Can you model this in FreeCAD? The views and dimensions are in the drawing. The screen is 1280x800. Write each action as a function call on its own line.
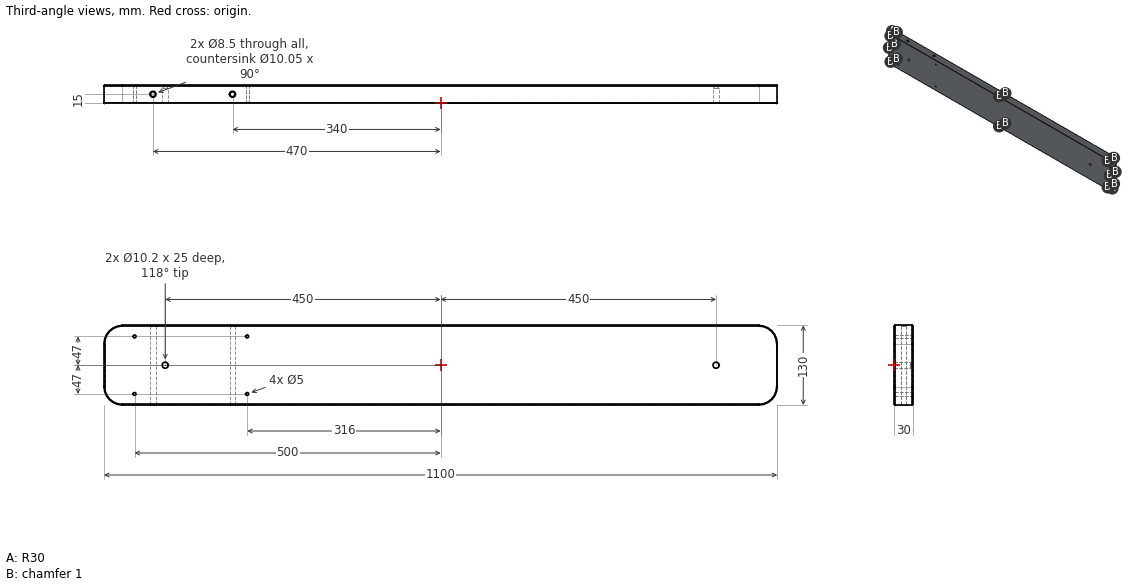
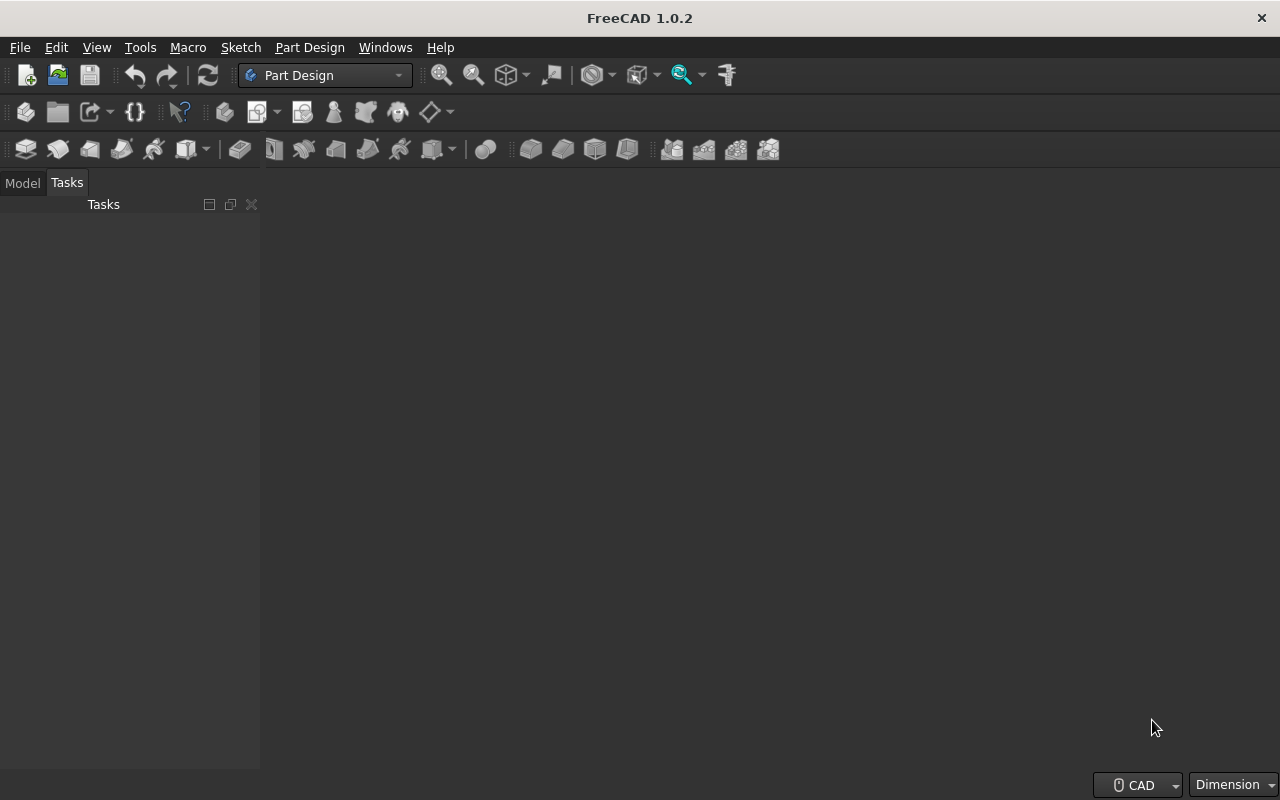
click(26, 76)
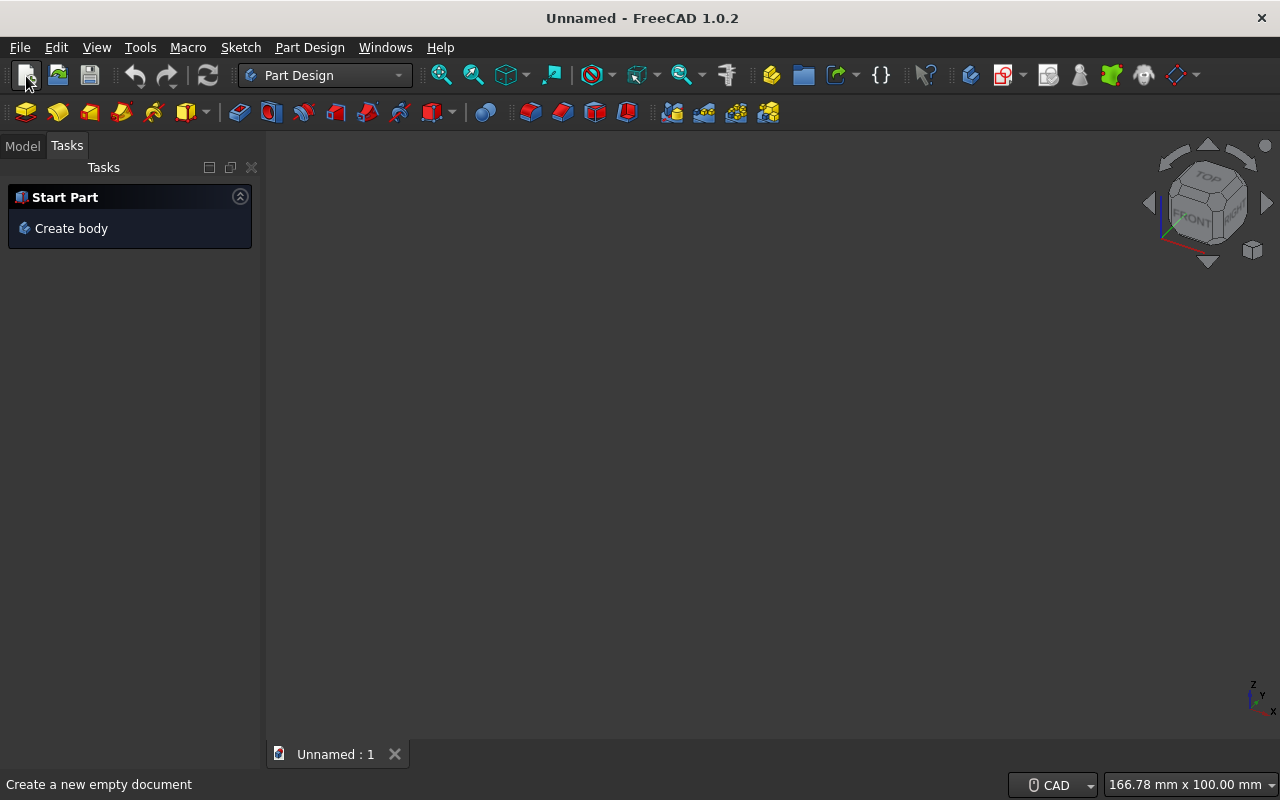
click(1004, 76)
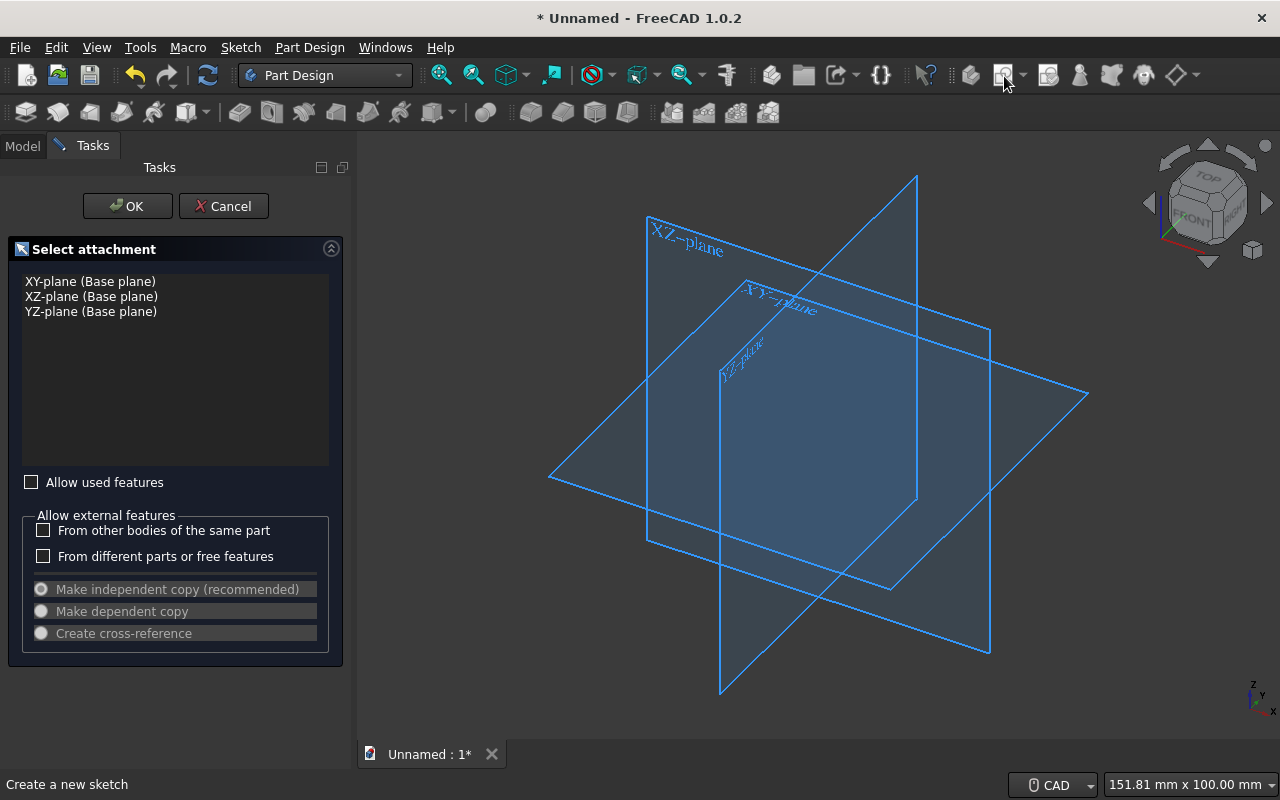
click(82, 296)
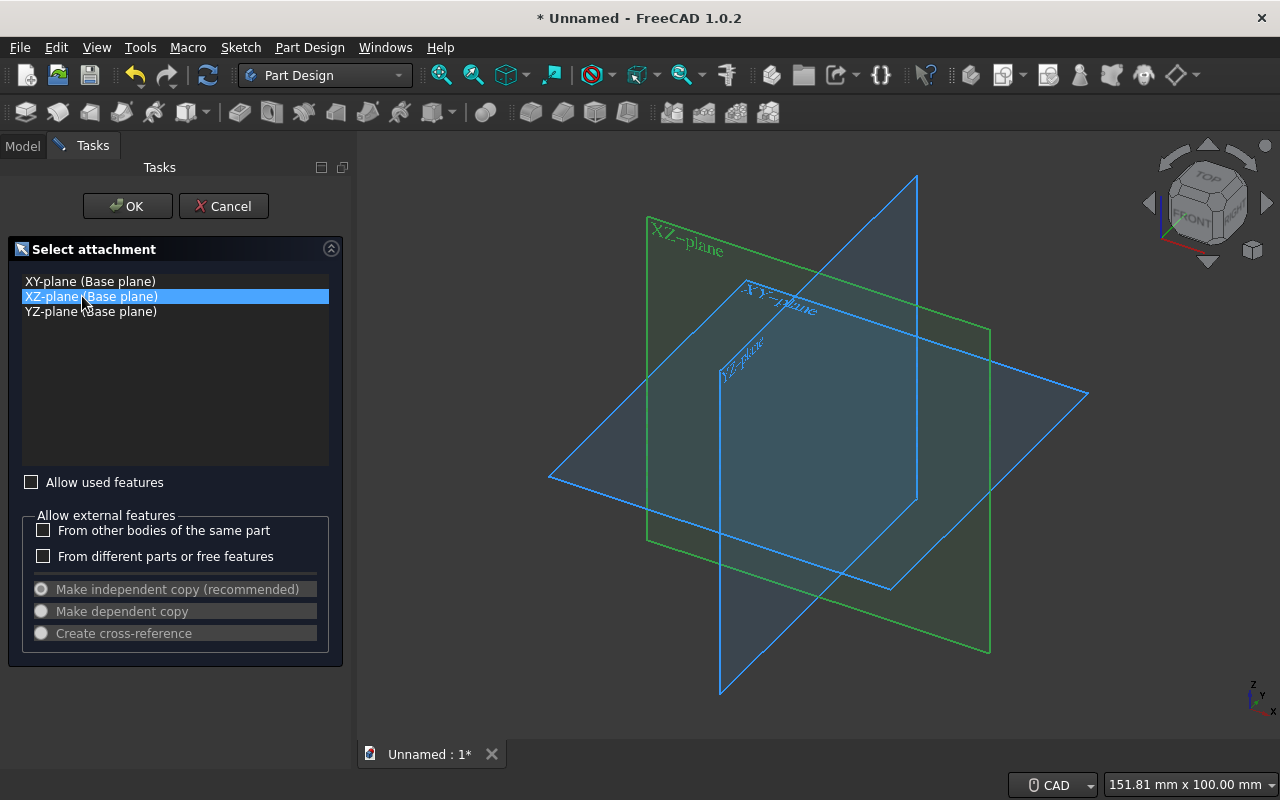
click(128, 206)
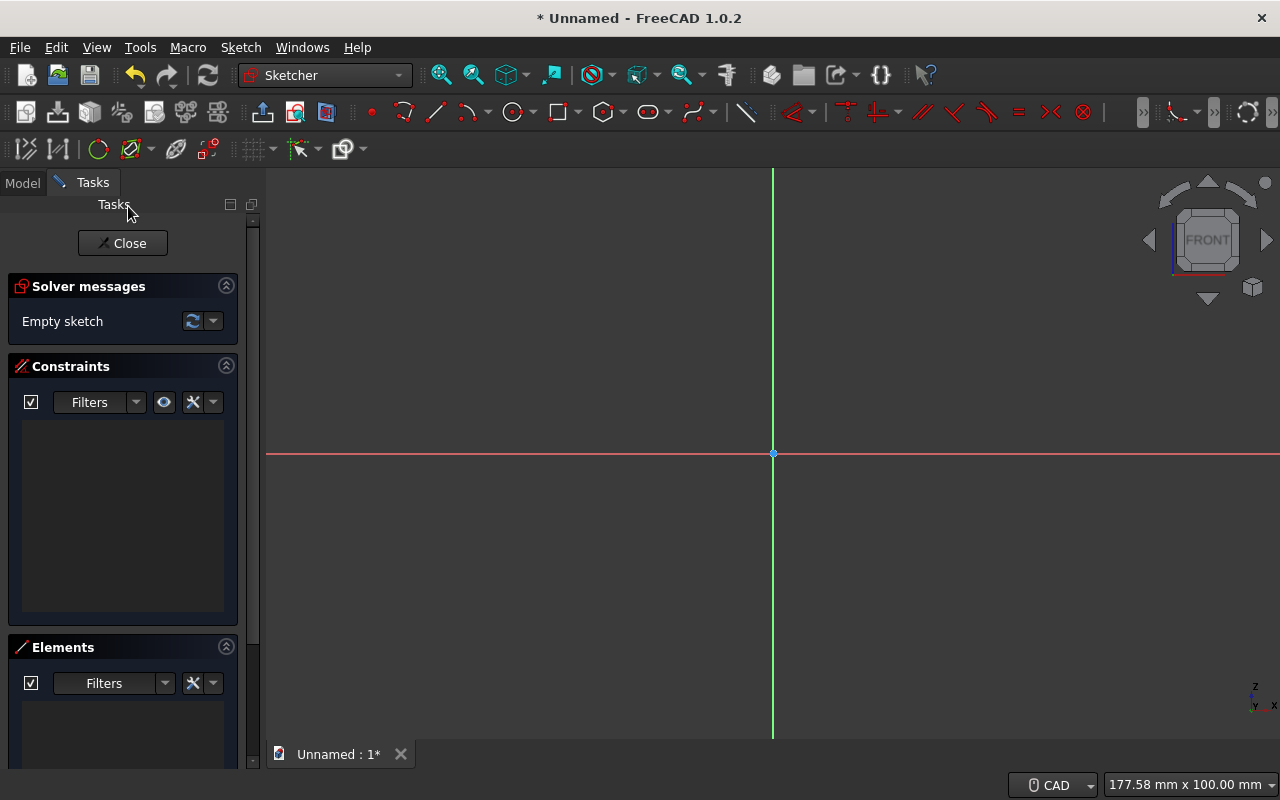
scroll(698, 454, down, 12)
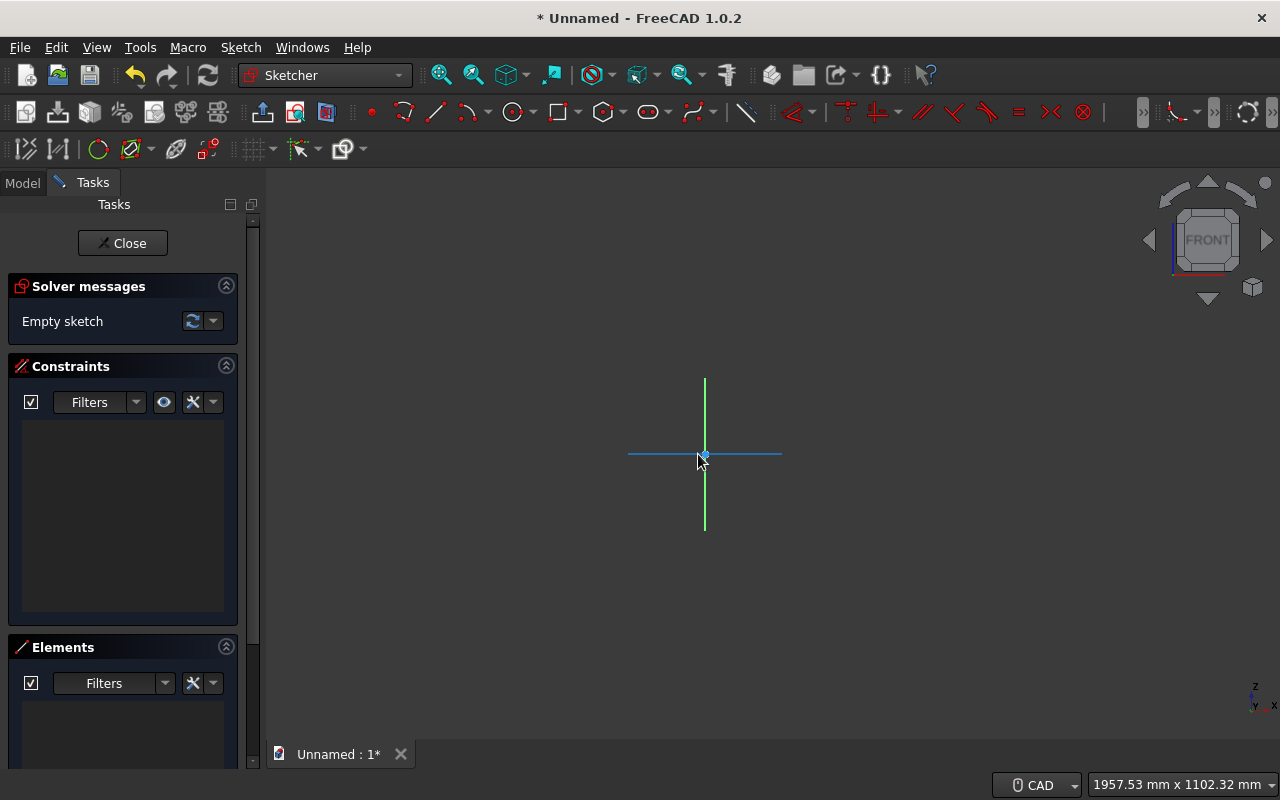
key(g)
key(v)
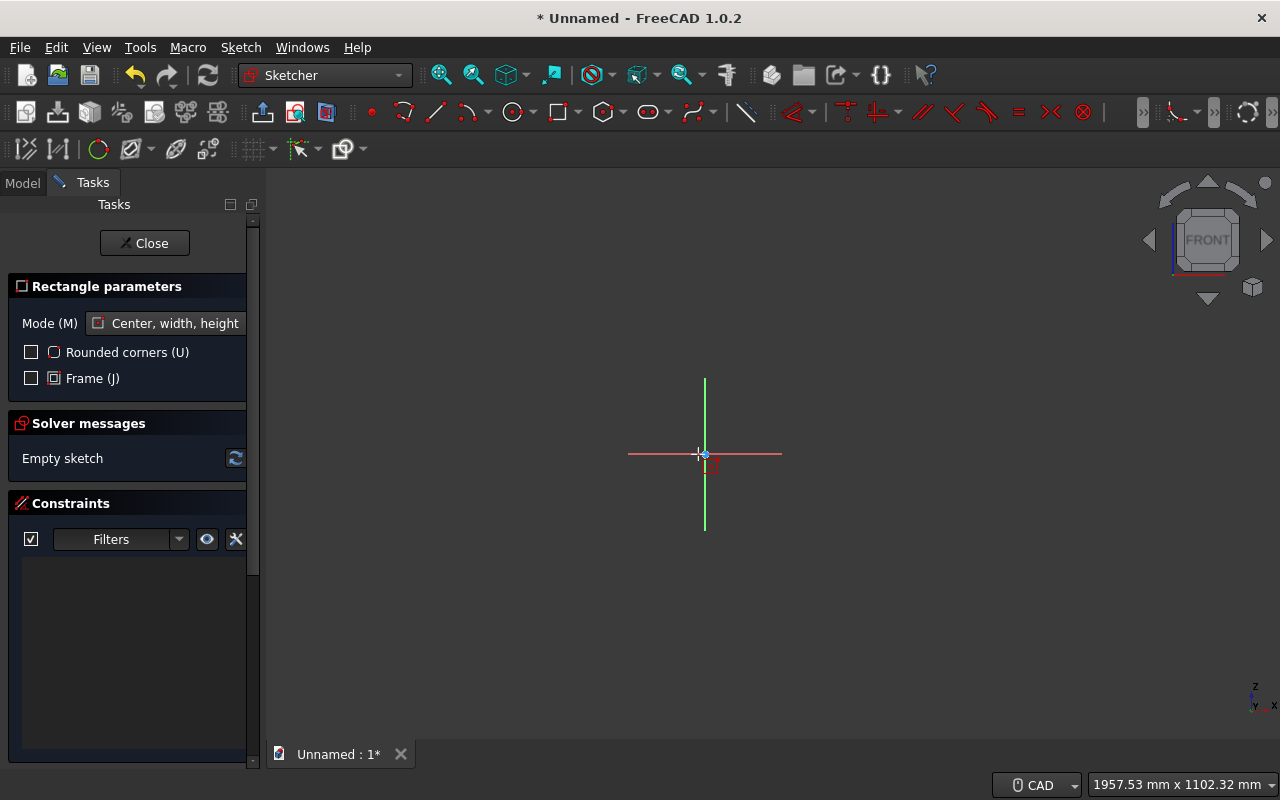
click(705, 454)
click(990, 421)
key(Escape)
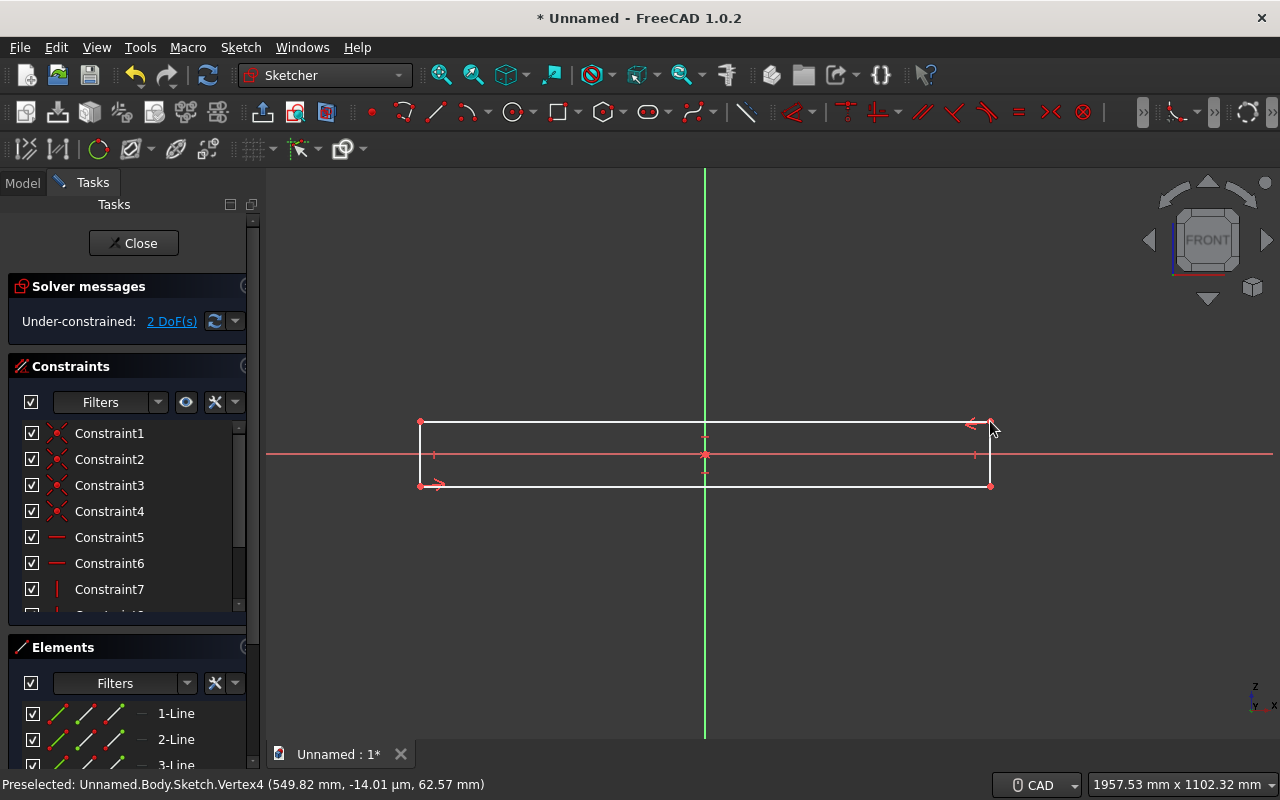
click(792, 112)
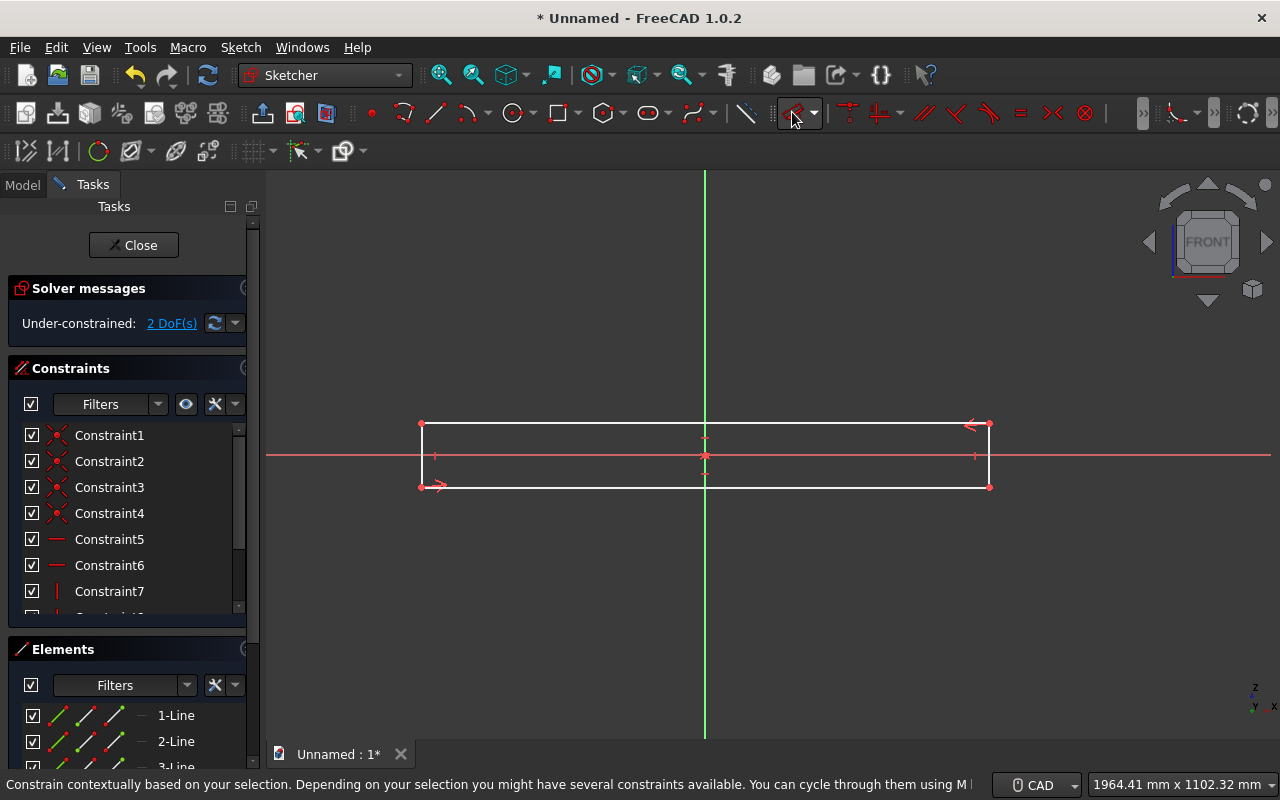
click(989, 468)
click(1023, 441)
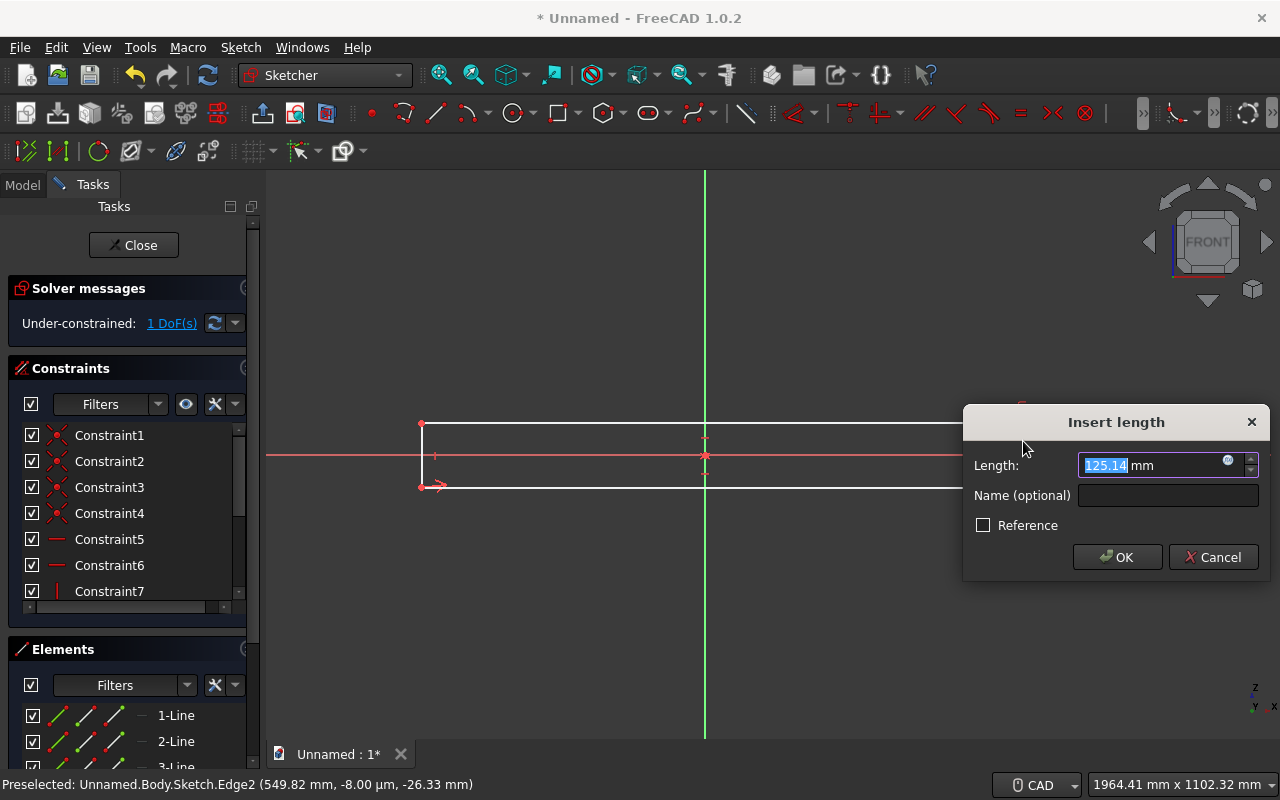
text(130)
key(Return)